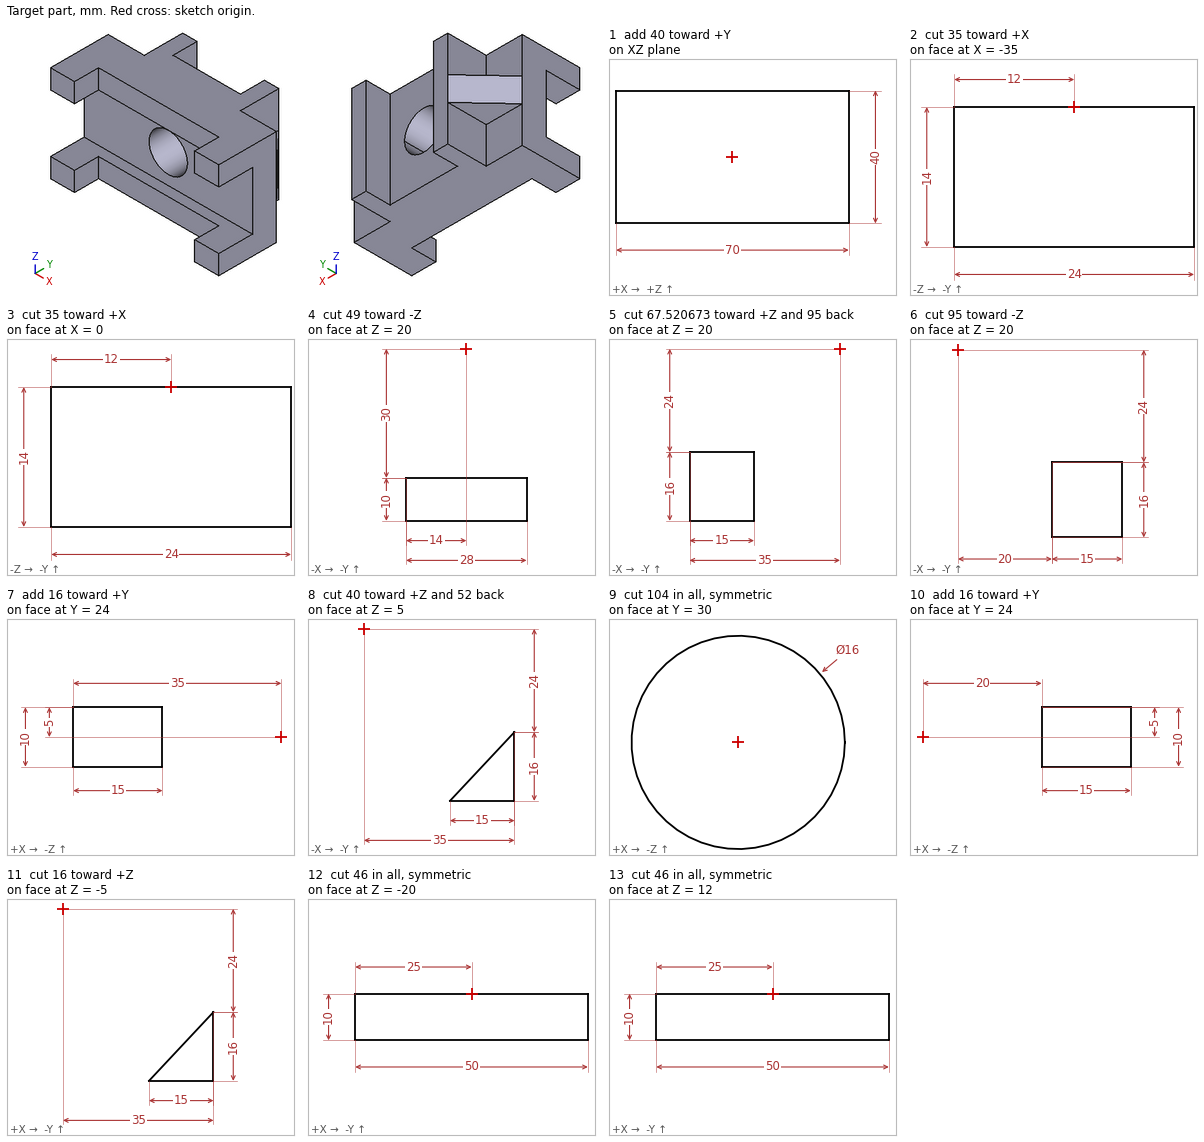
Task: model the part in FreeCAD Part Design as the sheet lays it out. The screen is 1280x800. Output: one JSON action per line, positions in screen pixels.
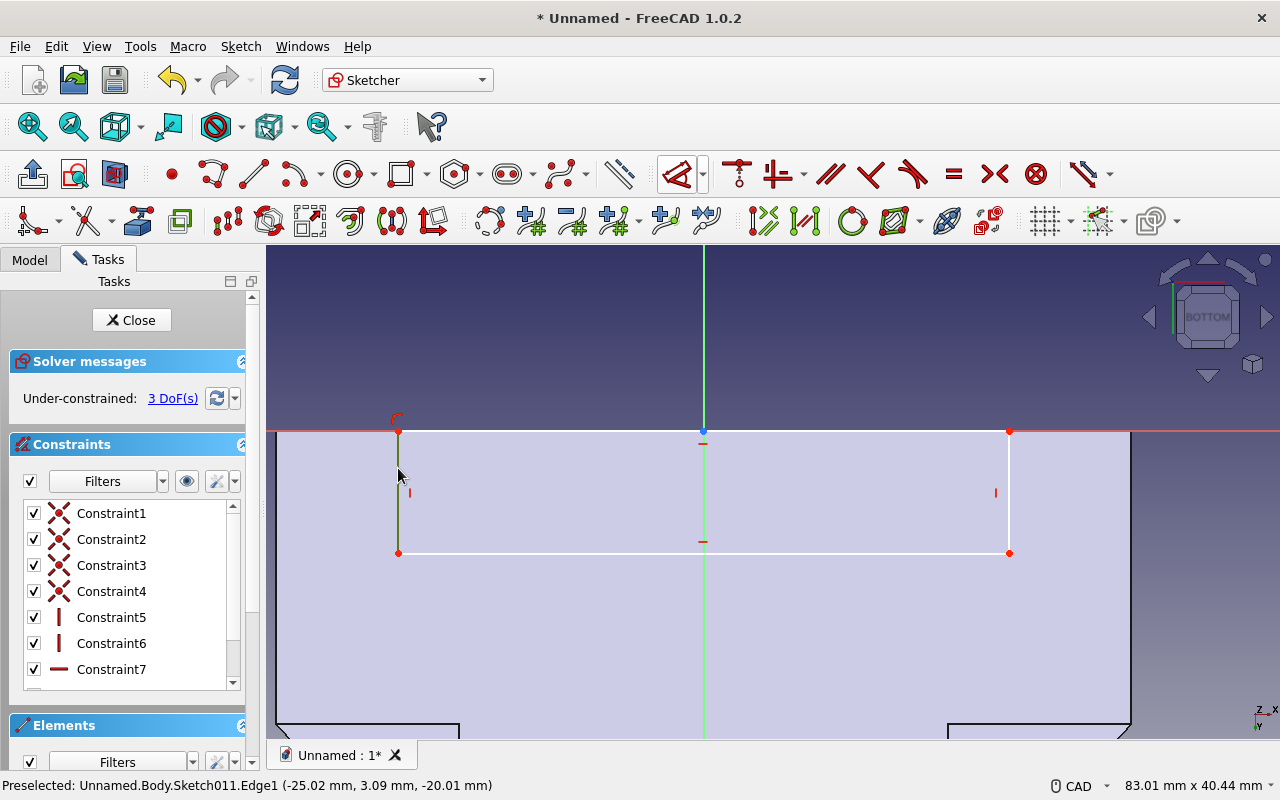
{"action": "left_click", "coordinate": [702, 174]}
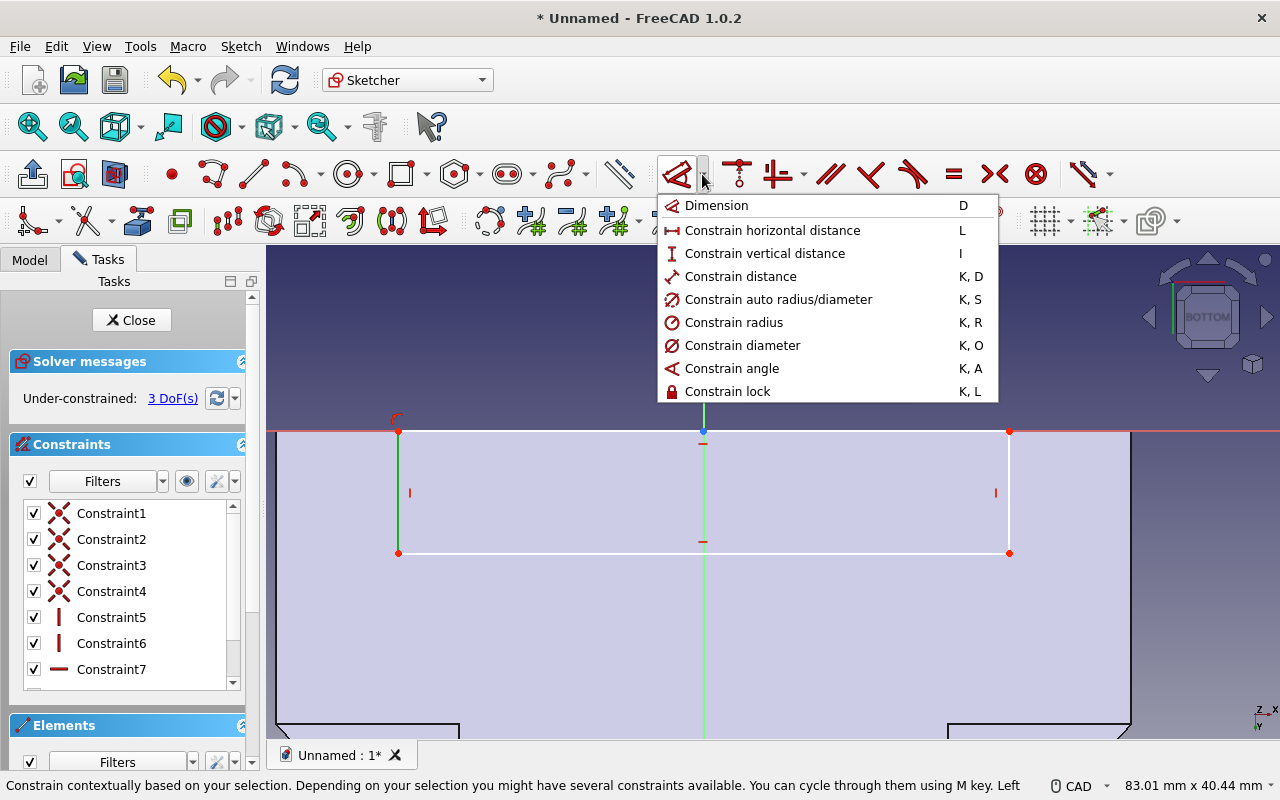
{"action": "left_click", "coordinate": [828, 254]}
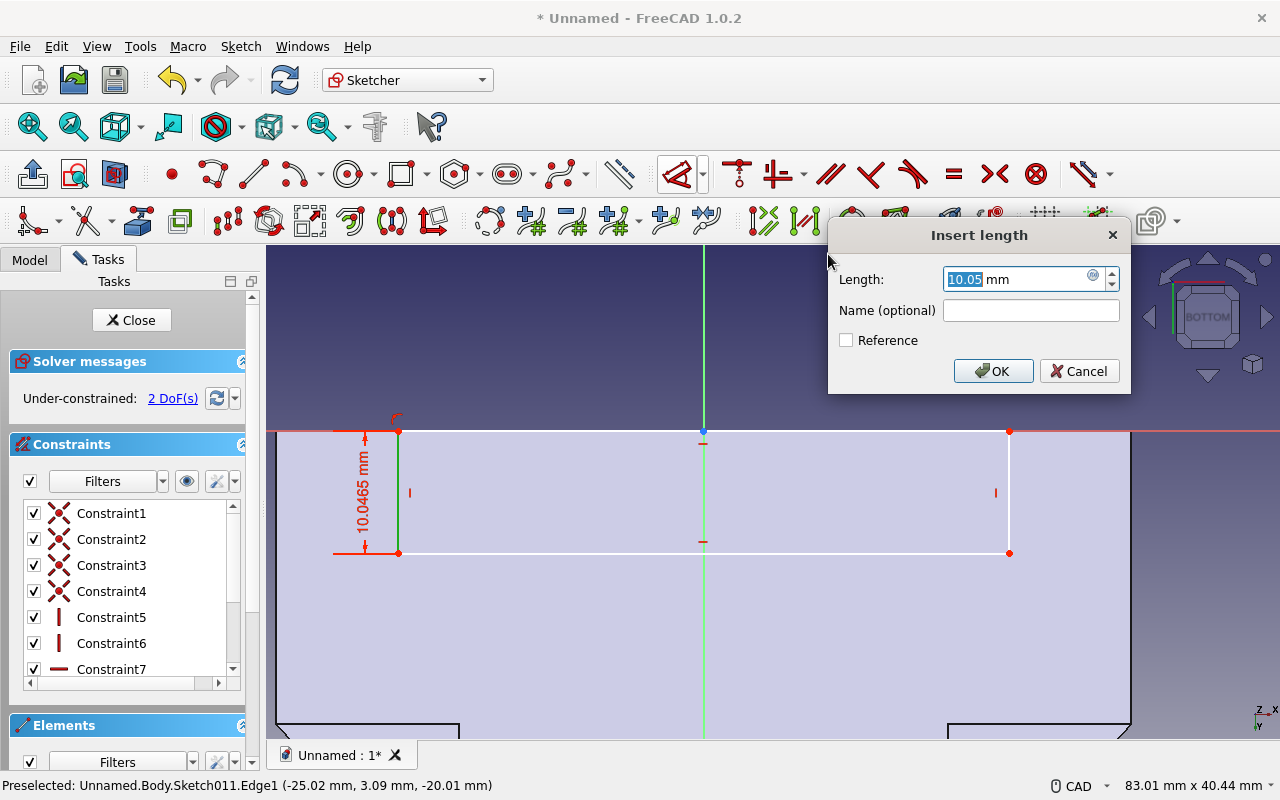
{"action": "type", "text": "10"}
{"action": "key", "text": "Return"}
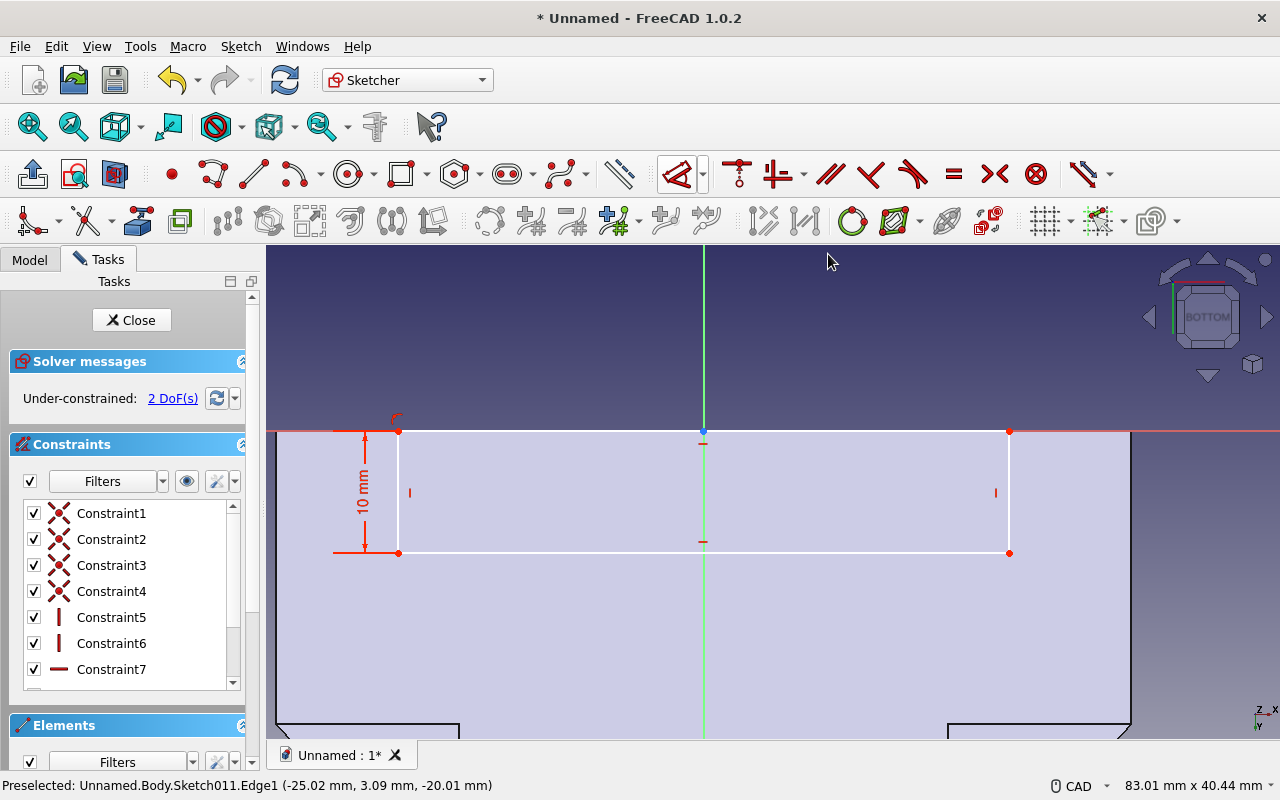
{"action": "left_click", "coordinate": [581, 553]}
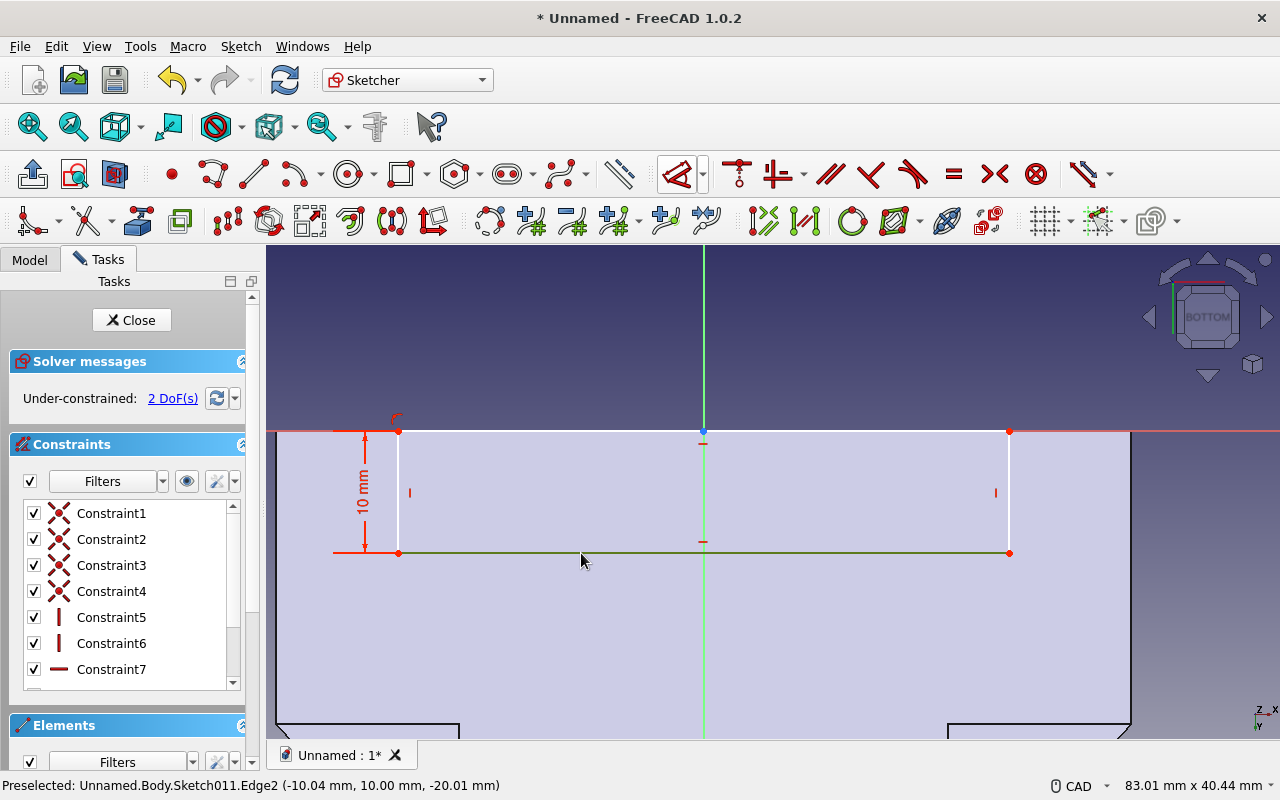
{"action": "key", "text": "l"}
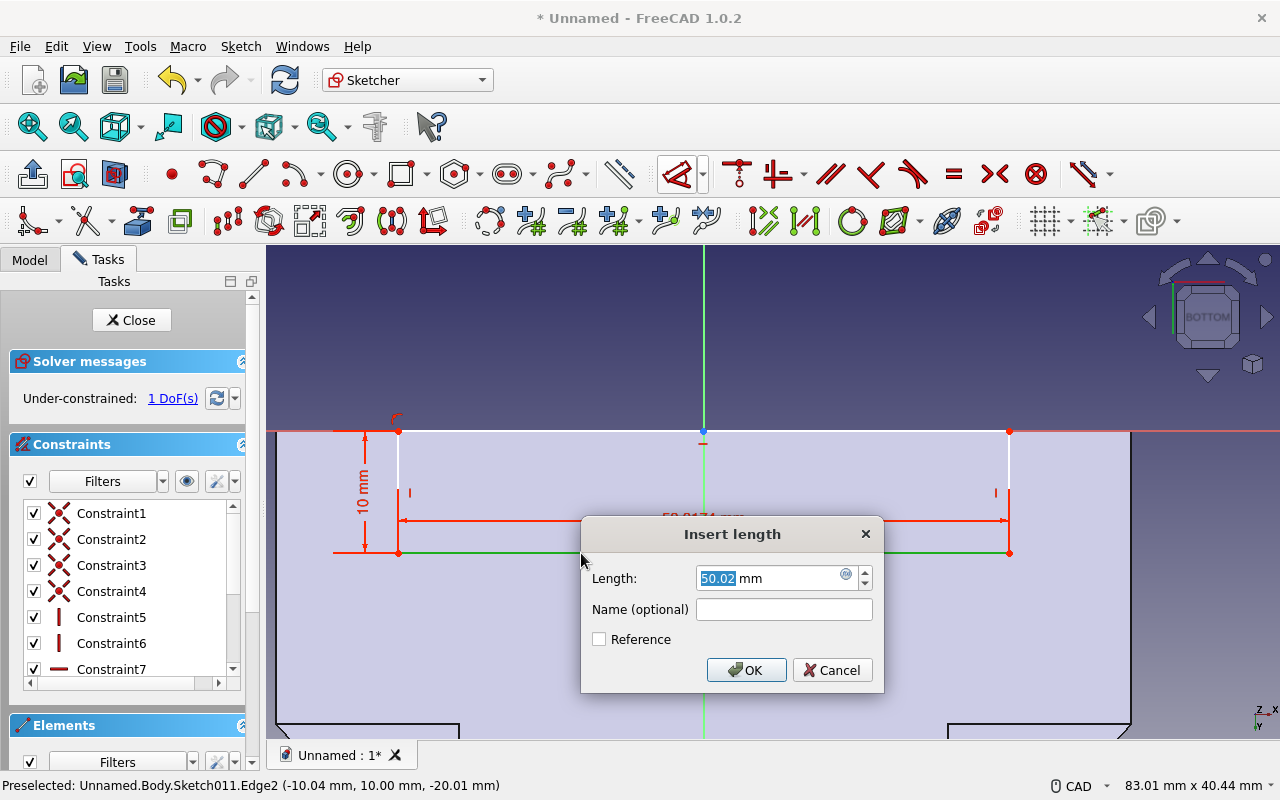
{"action": "type", "text": "50"}
{"action": "key", "text": "Return"}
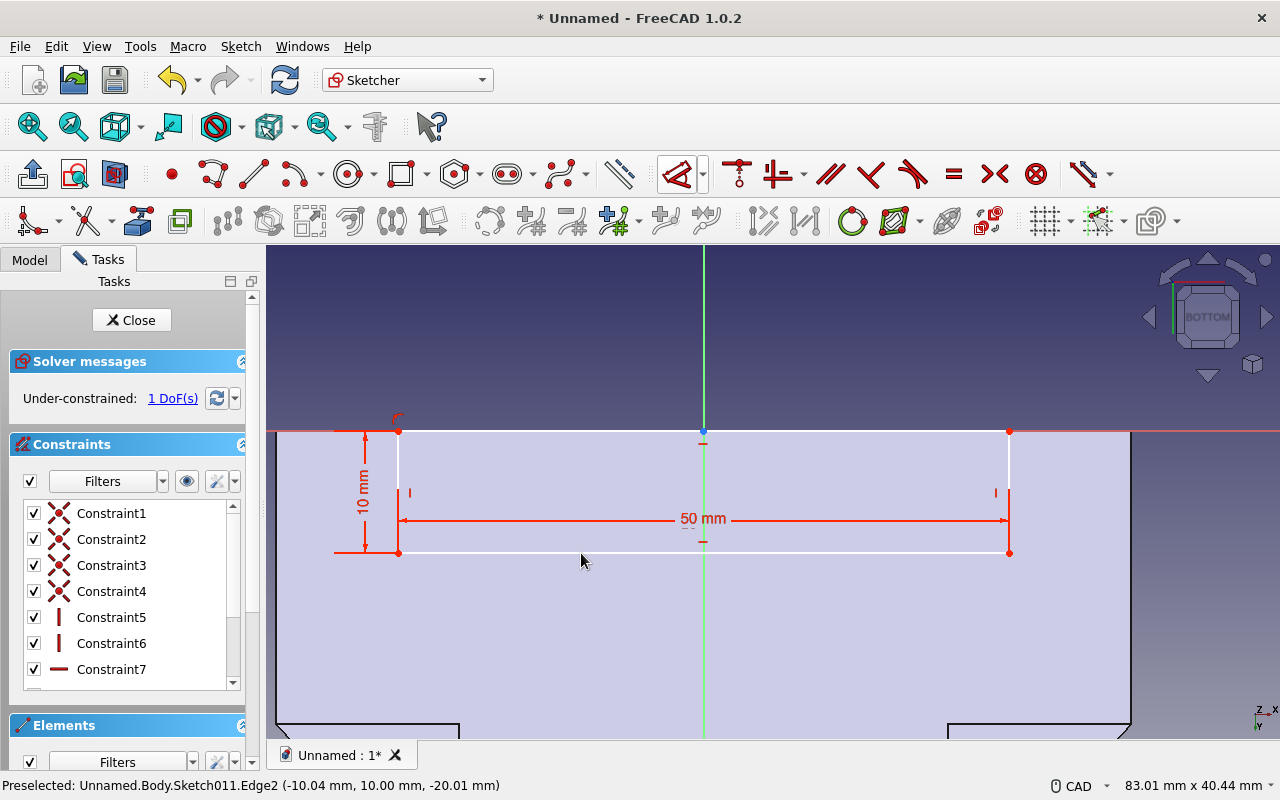
{"action": "left_click", "coordinate": [398, 431]}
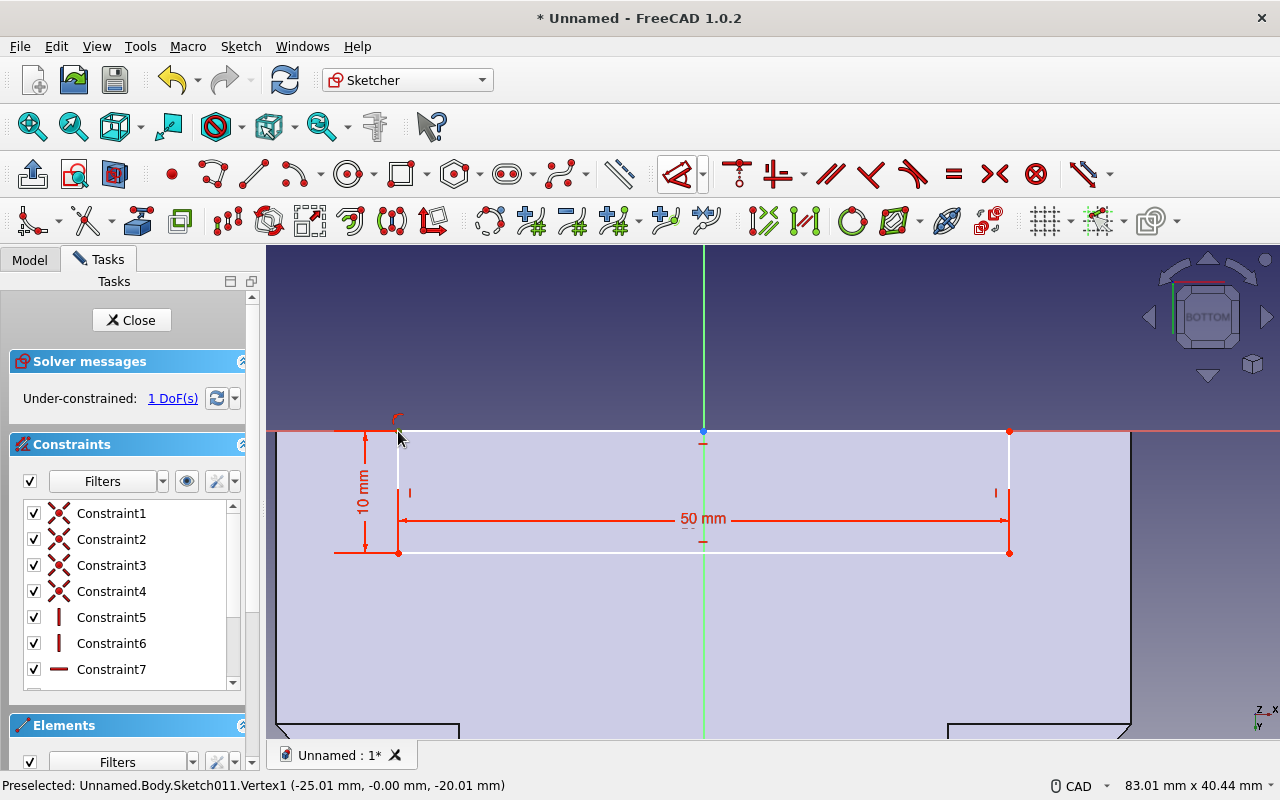
{"action": "key", "text": "l"}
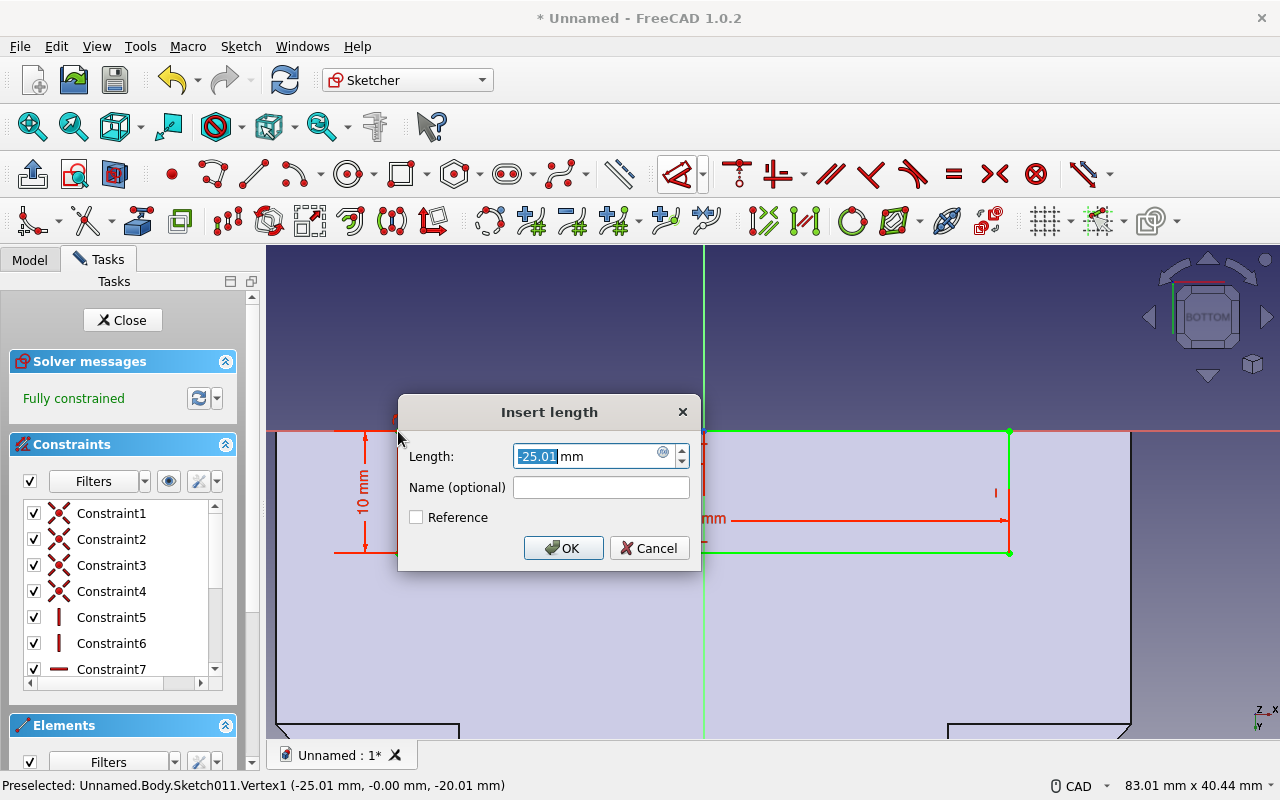
{"action": "type", "text": "-25"}
{"action": "key", "text": "Return"}